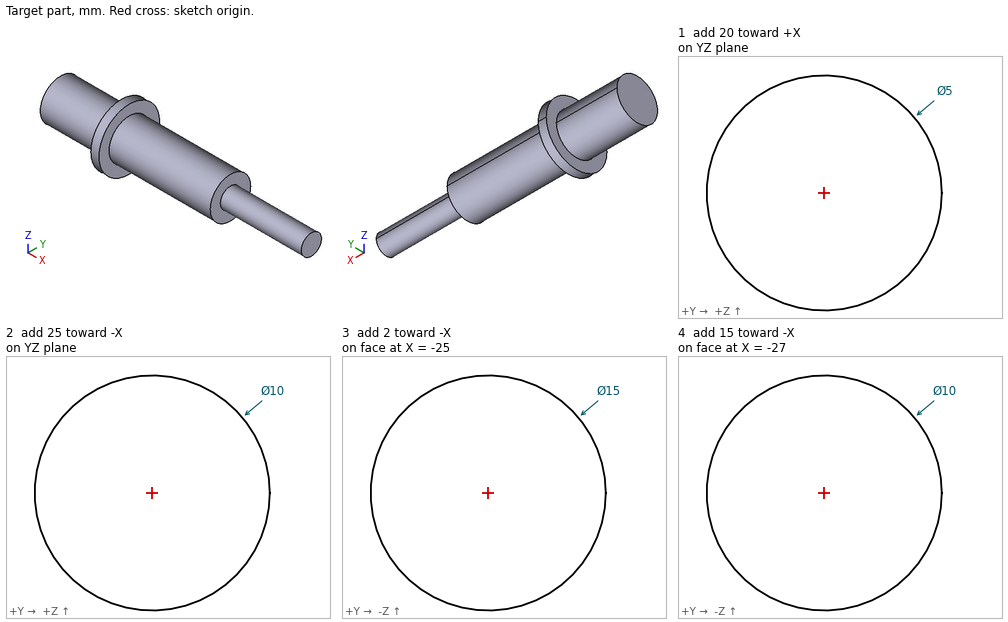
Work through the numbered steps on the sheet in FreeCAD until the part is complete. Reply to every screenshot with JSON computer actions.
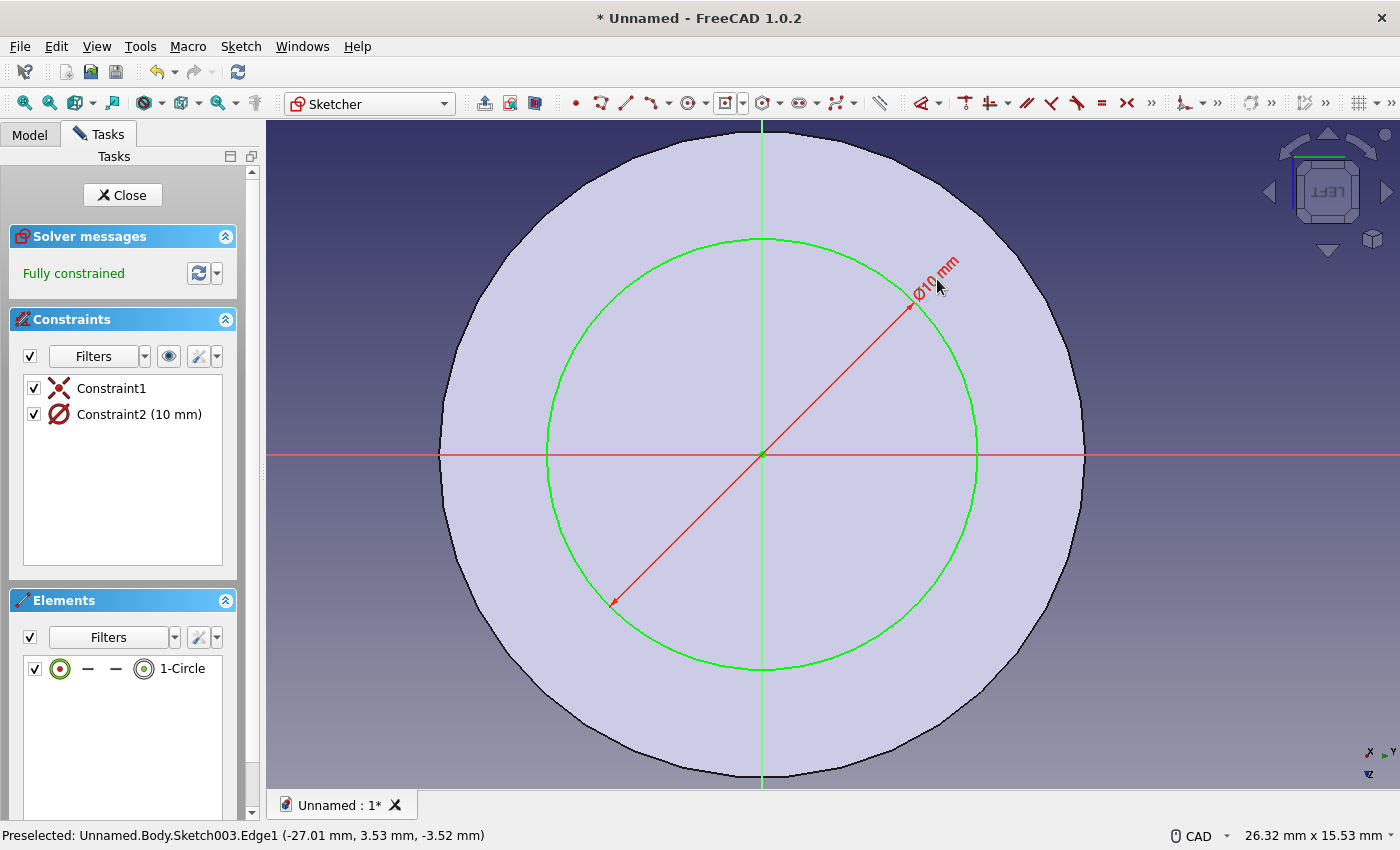
{"action": "left_click", "coordinate": [123, 195]}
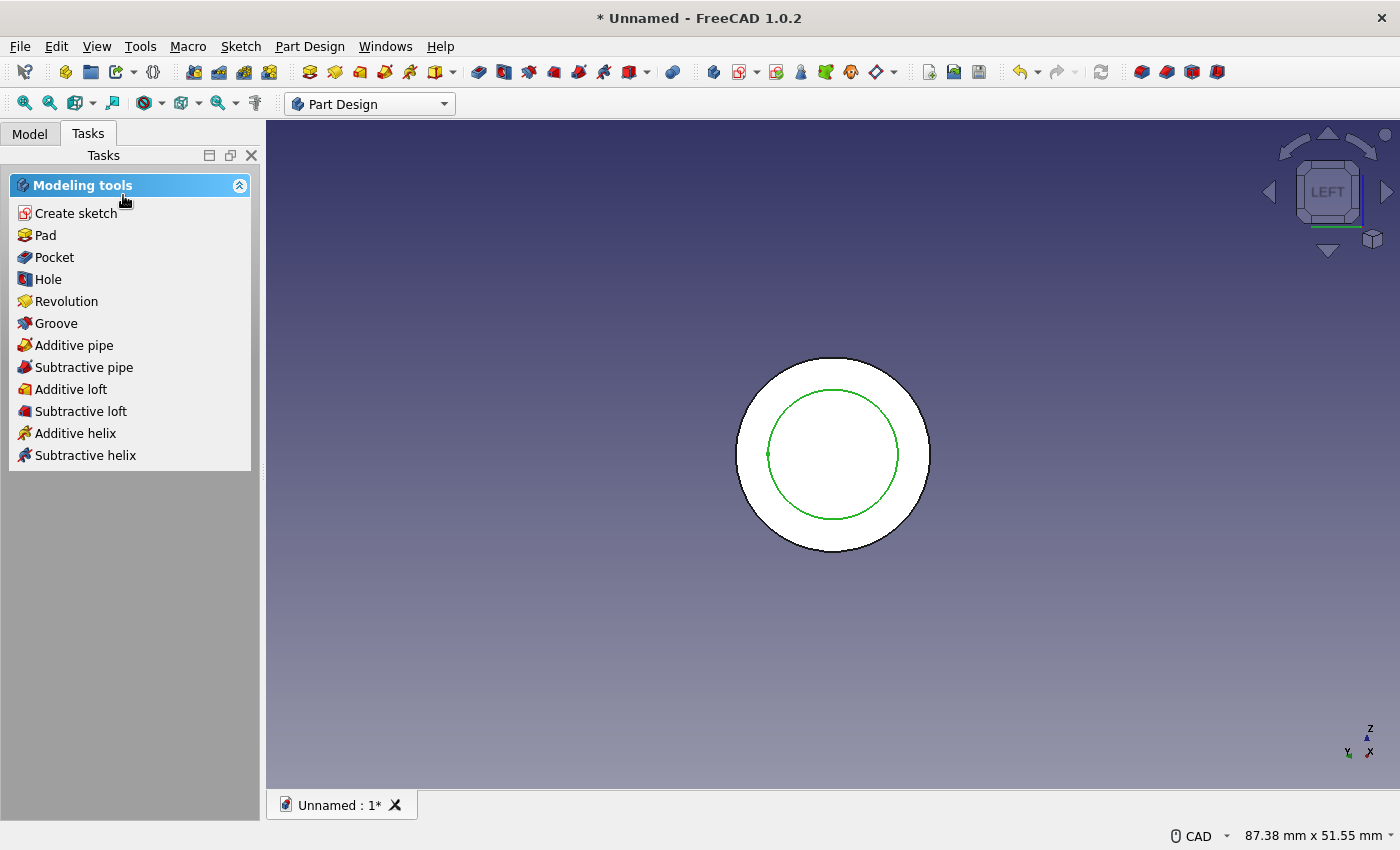
{"action": "left_click", "coordinate": [310, 72]}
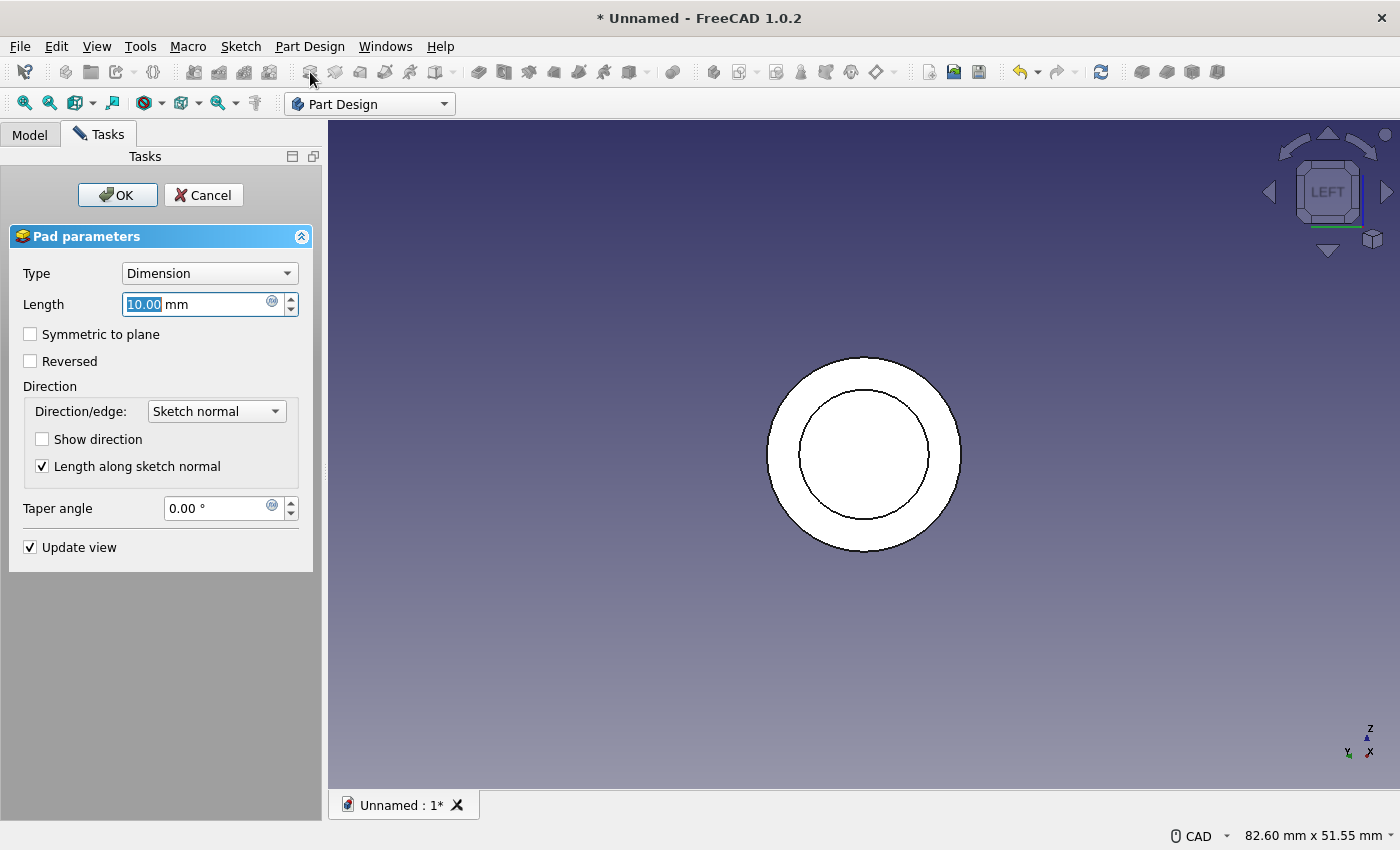
{"action": "type", "text": "15"}
{"action": "key", "text": "Tab"}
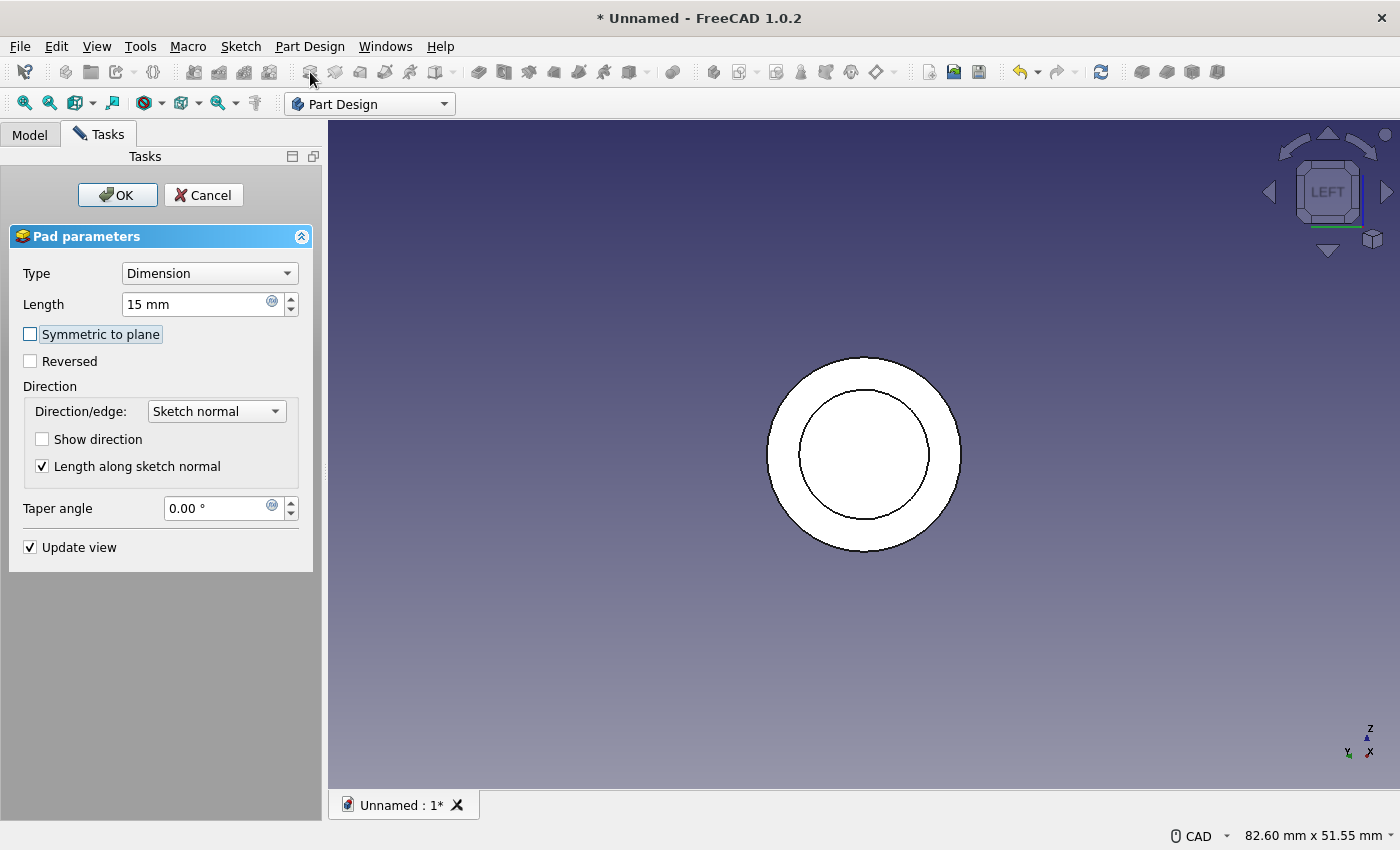
{"action": "left_click", "coordinate": [118, 195]}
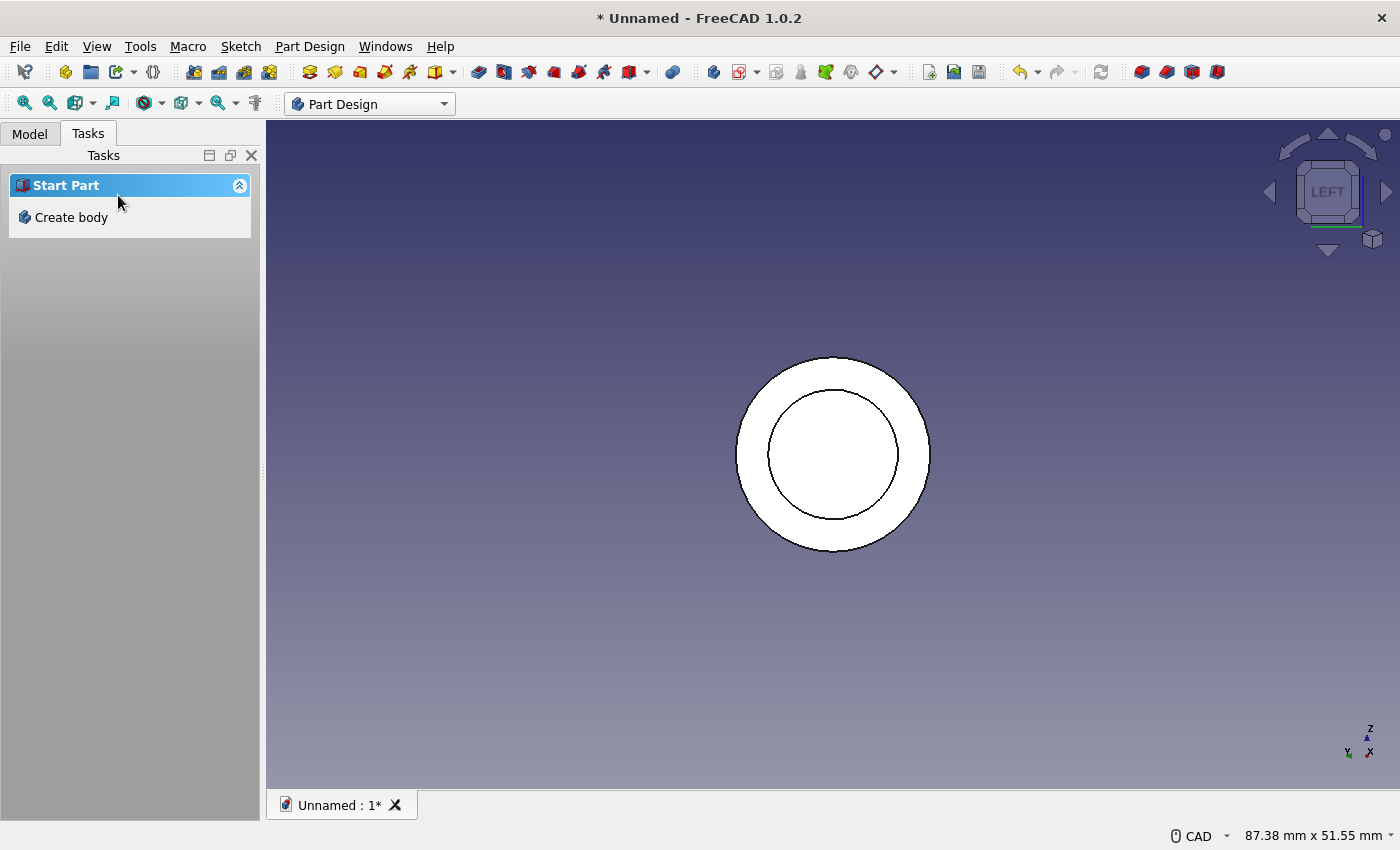
{"action": "key", "text": "0"}